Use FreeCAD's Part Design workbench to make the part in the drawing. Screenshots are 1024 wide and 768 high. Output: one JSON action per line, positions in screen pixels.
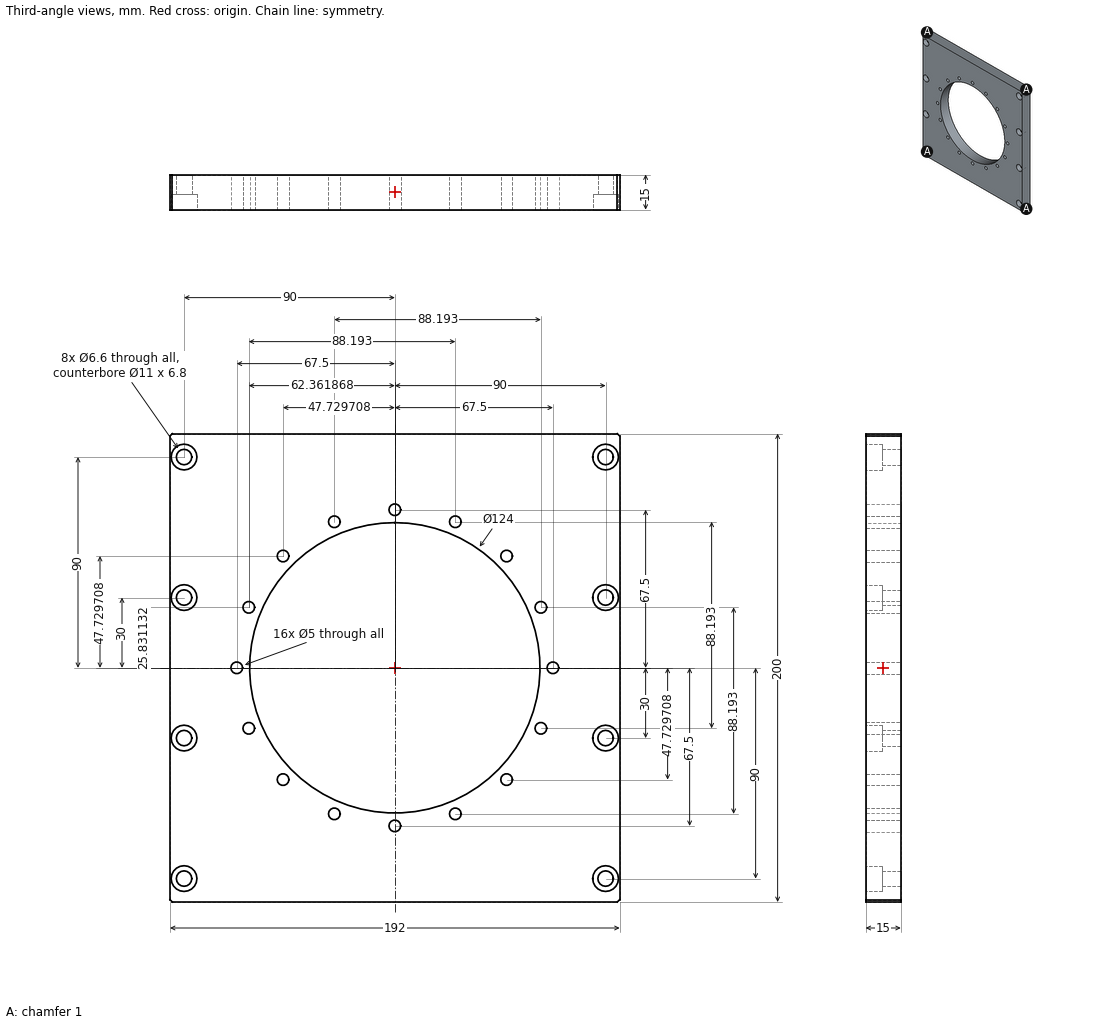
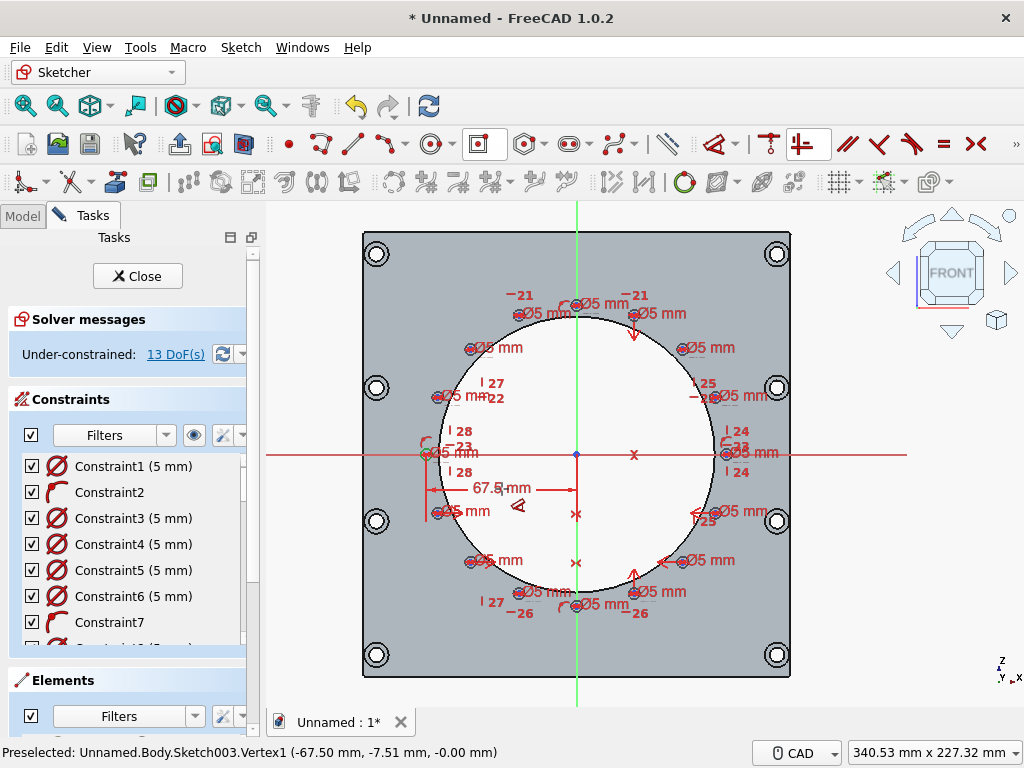
{"action": "left_click", "coordinate": [577, 306]}
{"action": "left_click", "coordinate": [611, 380]}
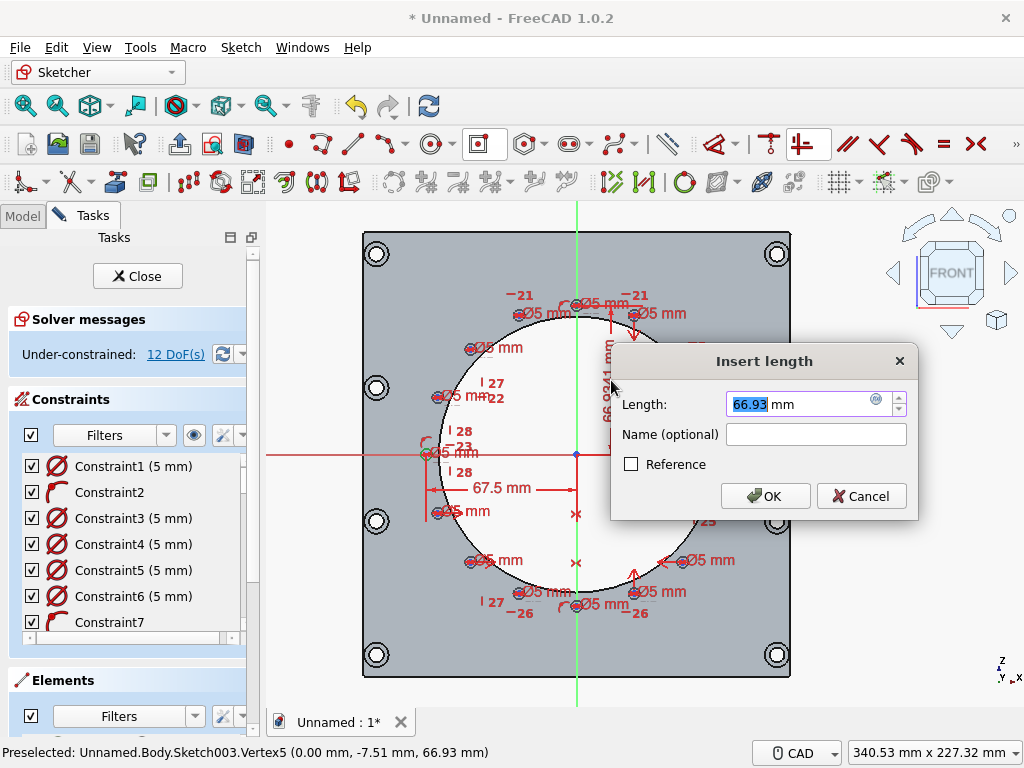
{"action": "type", "text": "67.5"}
{"action": "key", "text": "Return"}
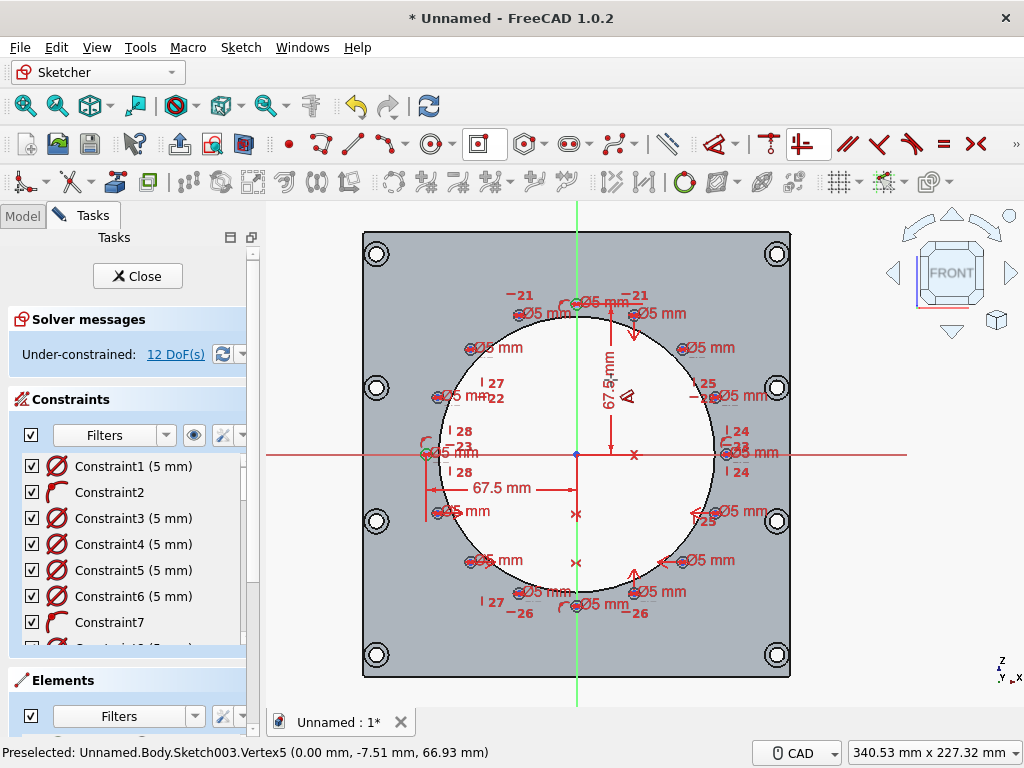
{"action": "left_click", "coordinate": [727, 455]}
{"action": "left_click", "coordinate": [652, 489]}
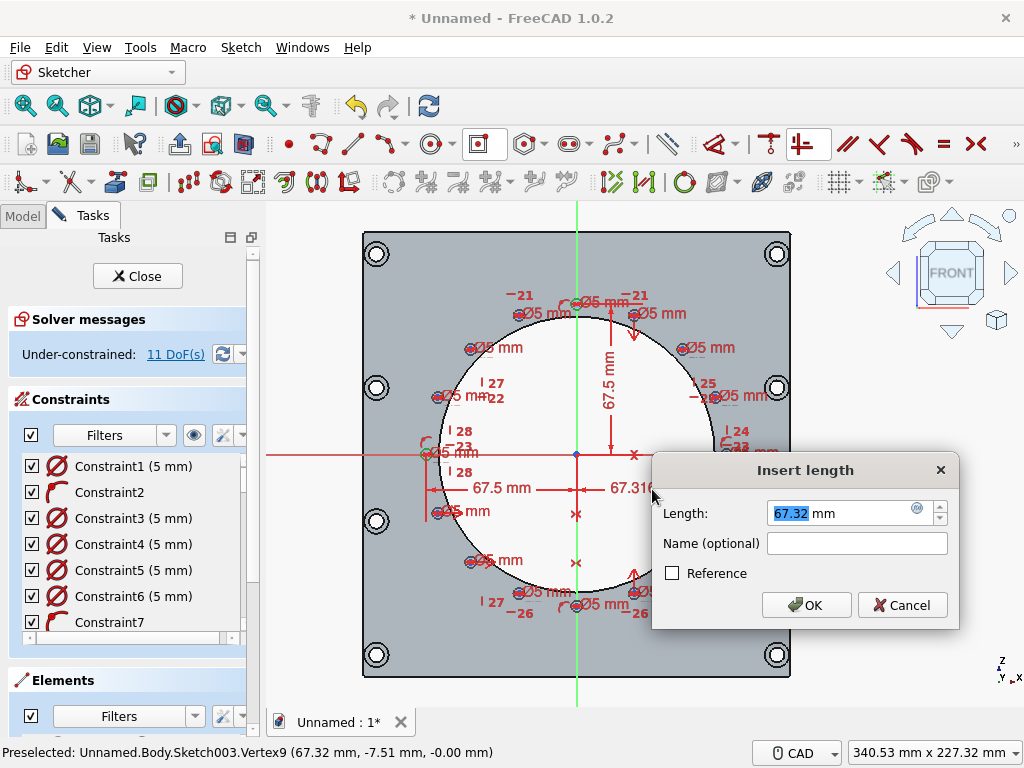
{"action": "type", "text": "67.5"}
{"action": "key", "text": "Return"}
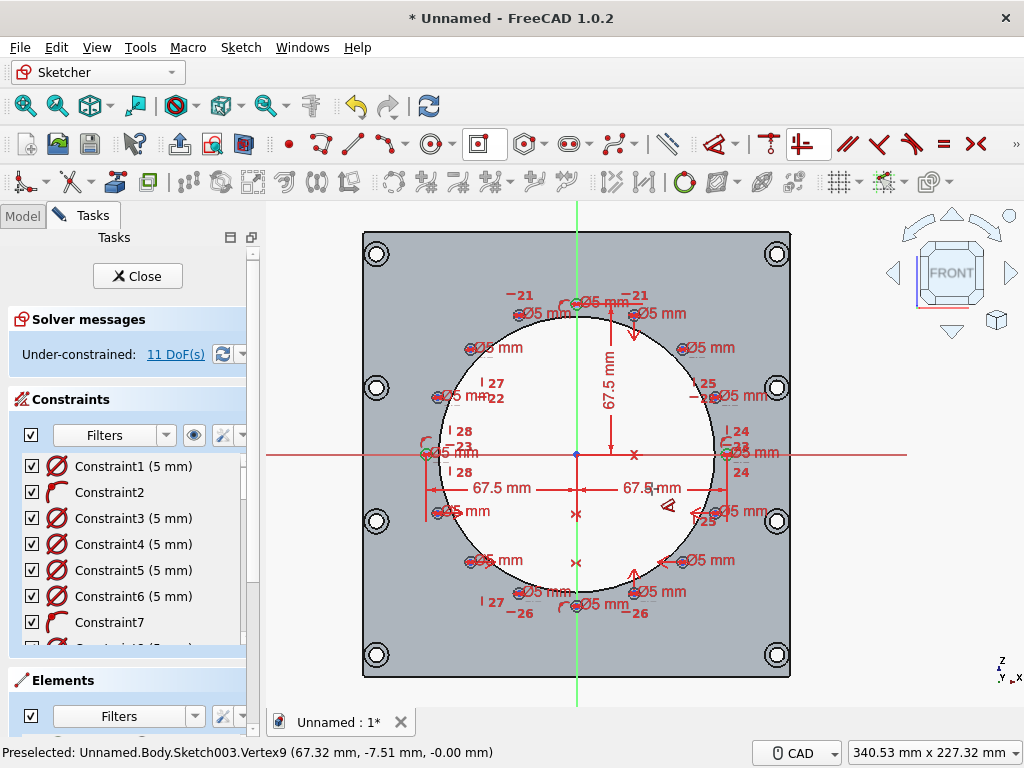
{"action": "left_click", "coordinate": [577, 606]}
{"action": "left_click", "coordinate": [611, 530]}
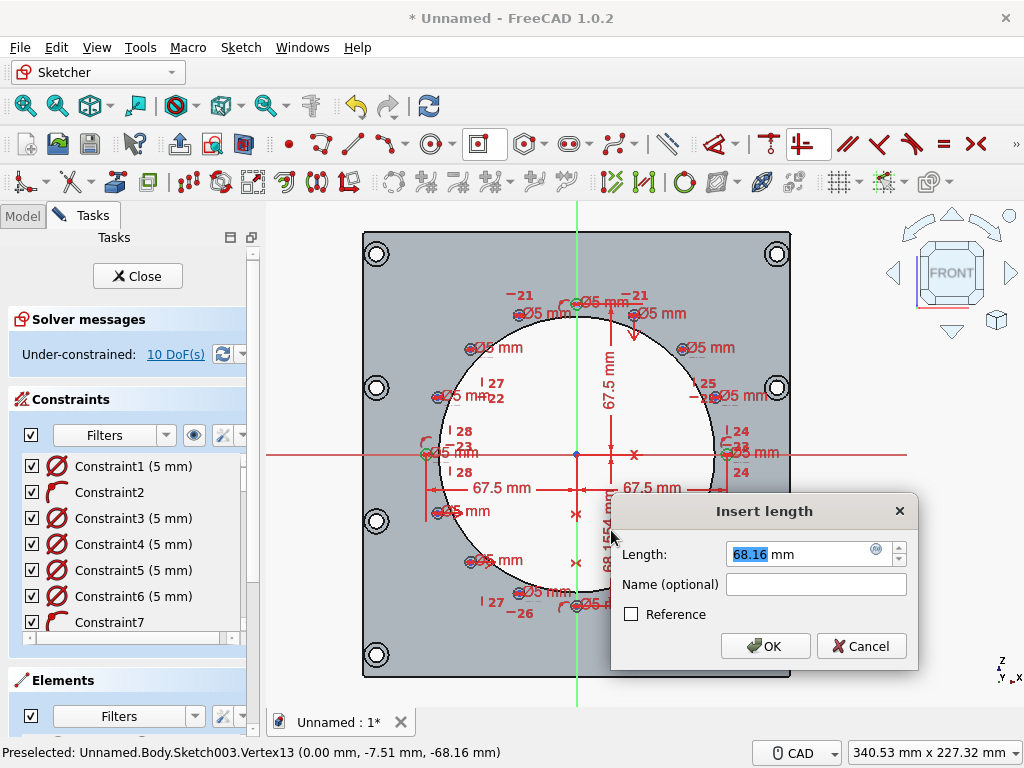
{"action": "type", "text": "67.5"}
{"action": "key", "text": "Return"}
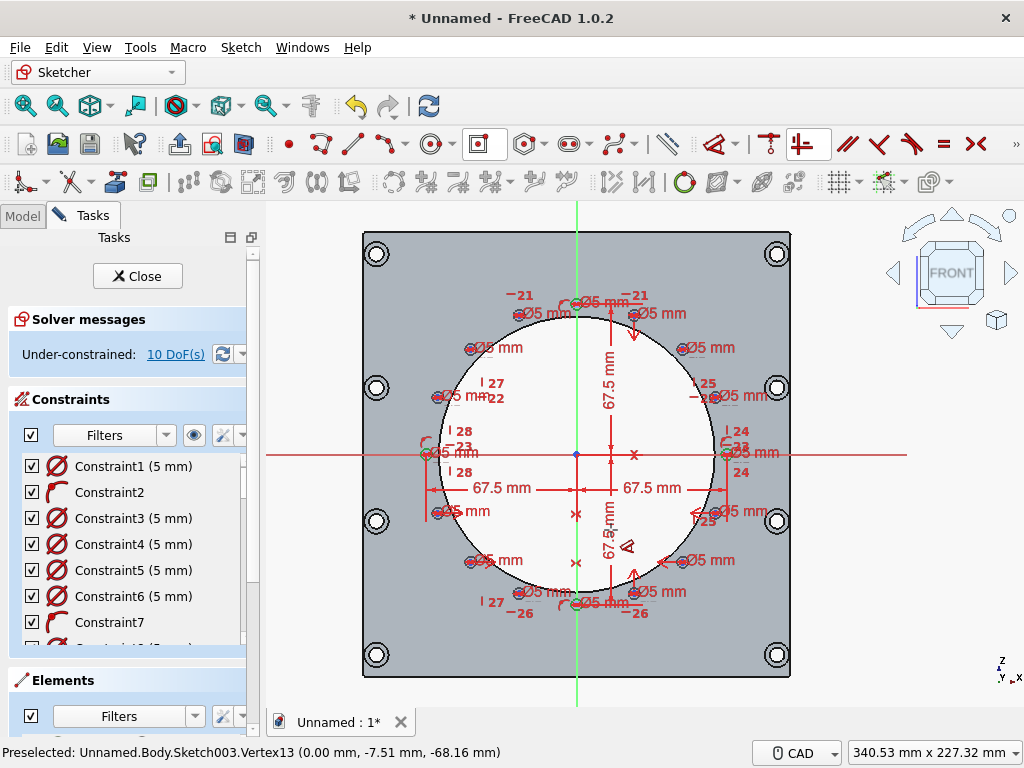
{"action": "left_click", "coordinate": [438, 398]}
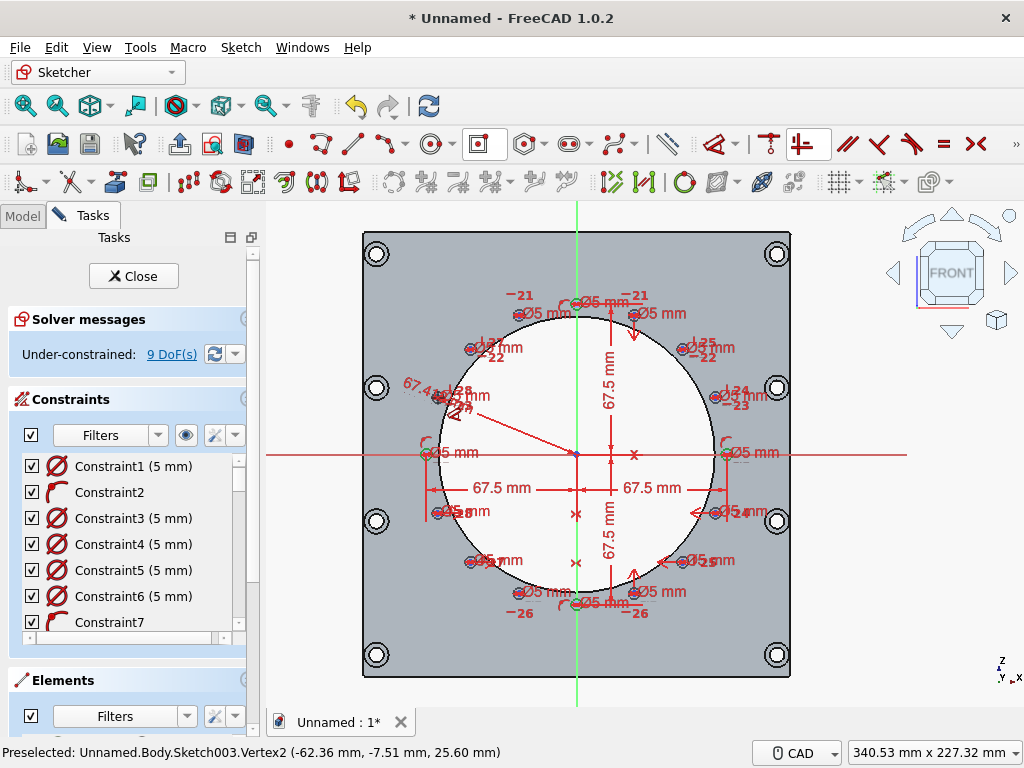
{"action": "left_click", "coordinate": [634, 315]}
{"action": "left_click", "coordinate": [536, 281]}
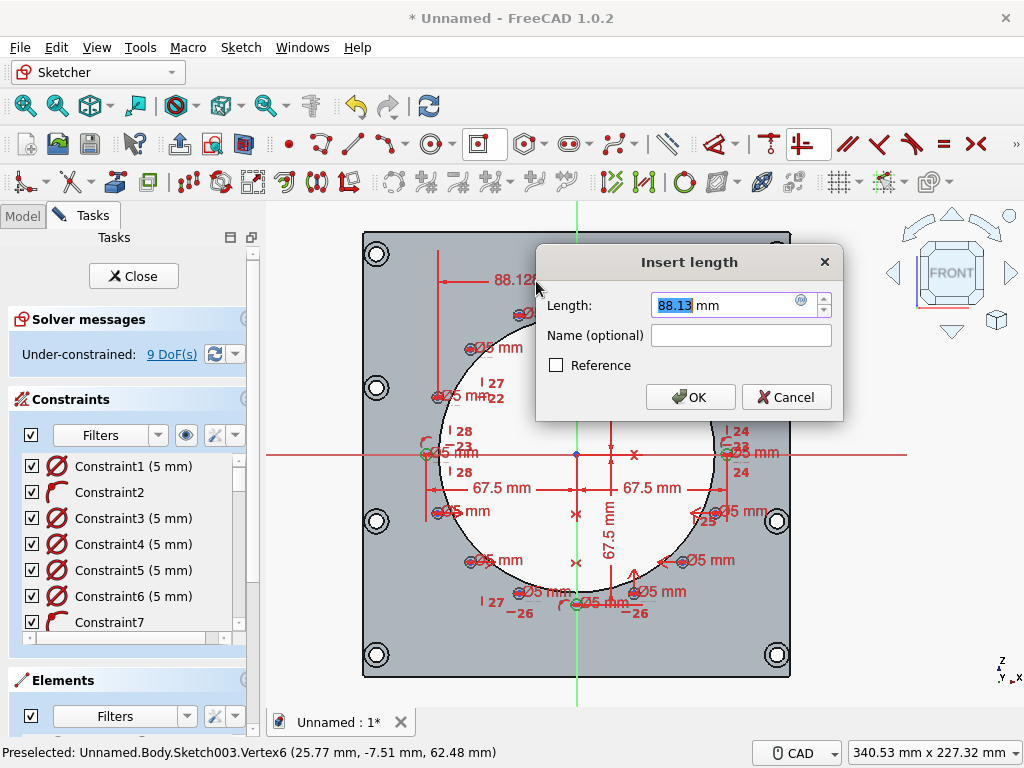
{"action": "type", "text": "88.193"}
{"action": "key", "text": "Return"}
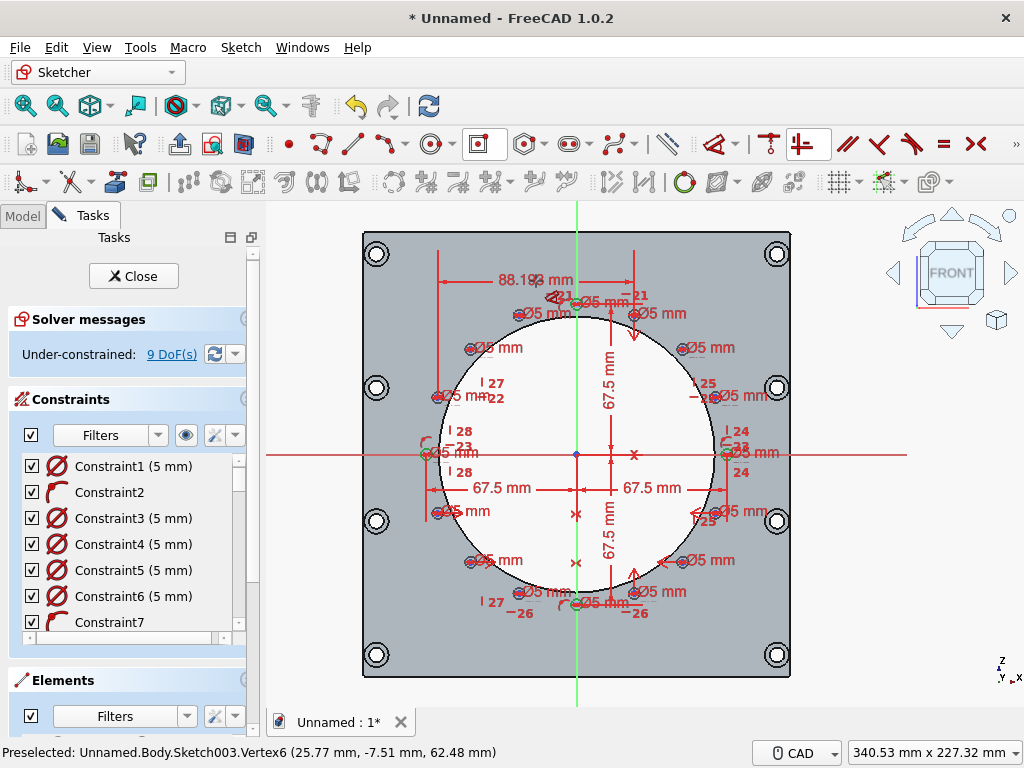
{"action": "left_click", "coordinate": [519, 315]}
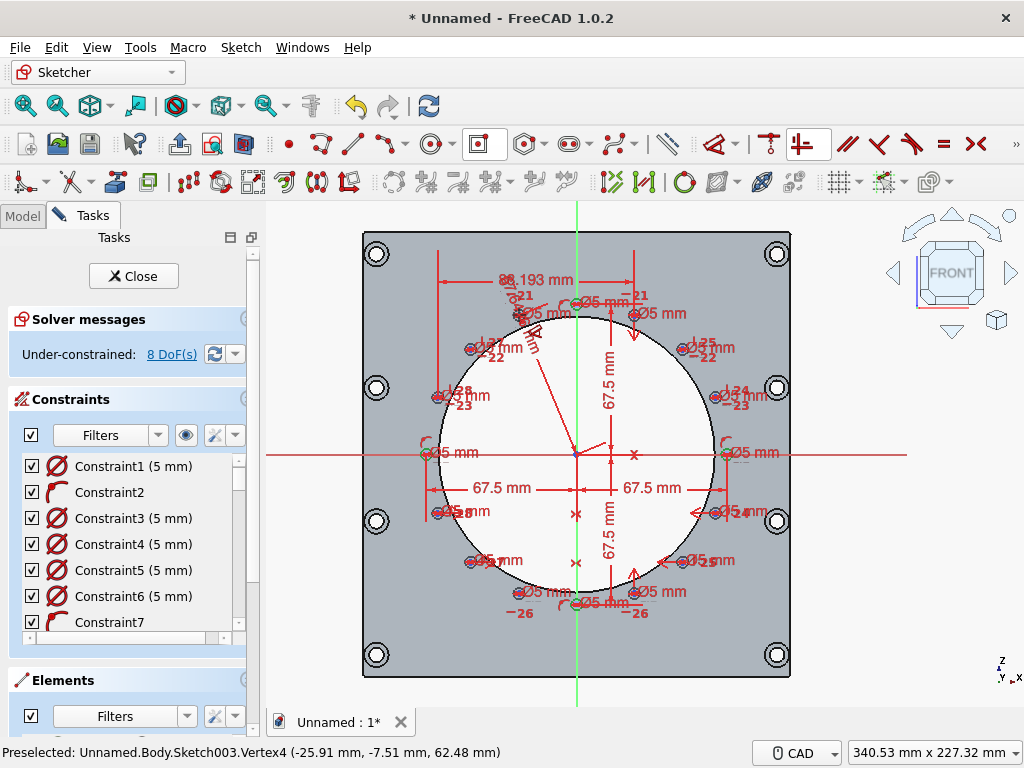
{"action": "left_click", "coordinate": [716, 398]}
{"action": "left_click", "coordinate": [617, 281]}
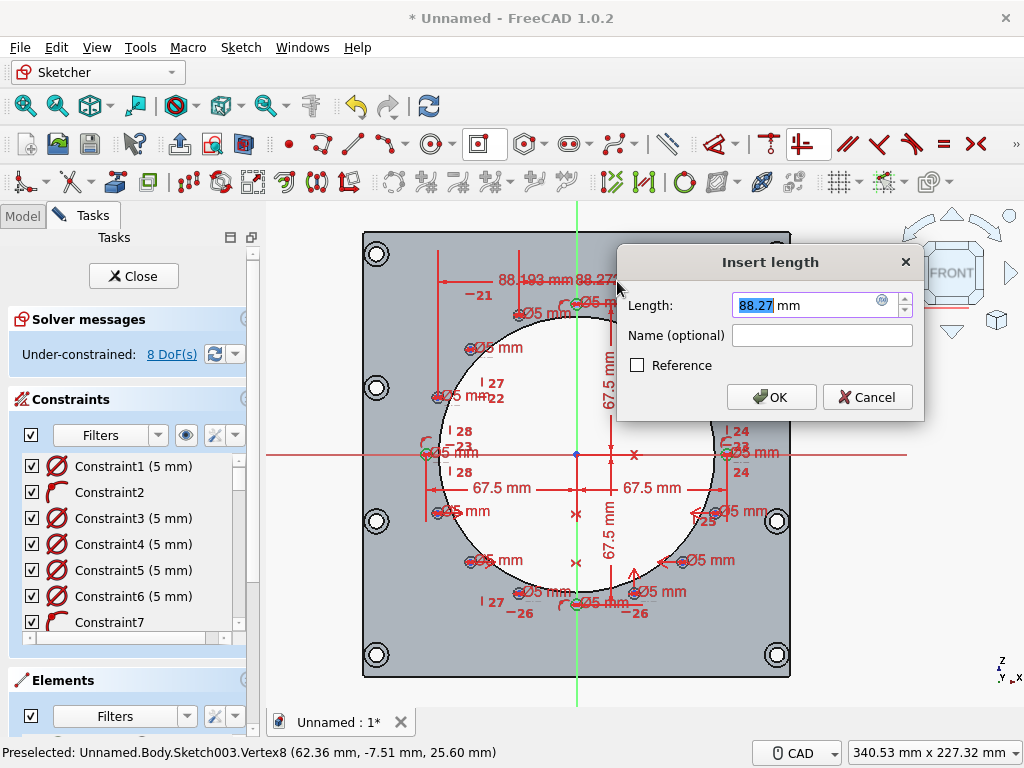
{"action": "type", "text": "88.193"}
{"action": "key", "text": "Return"}